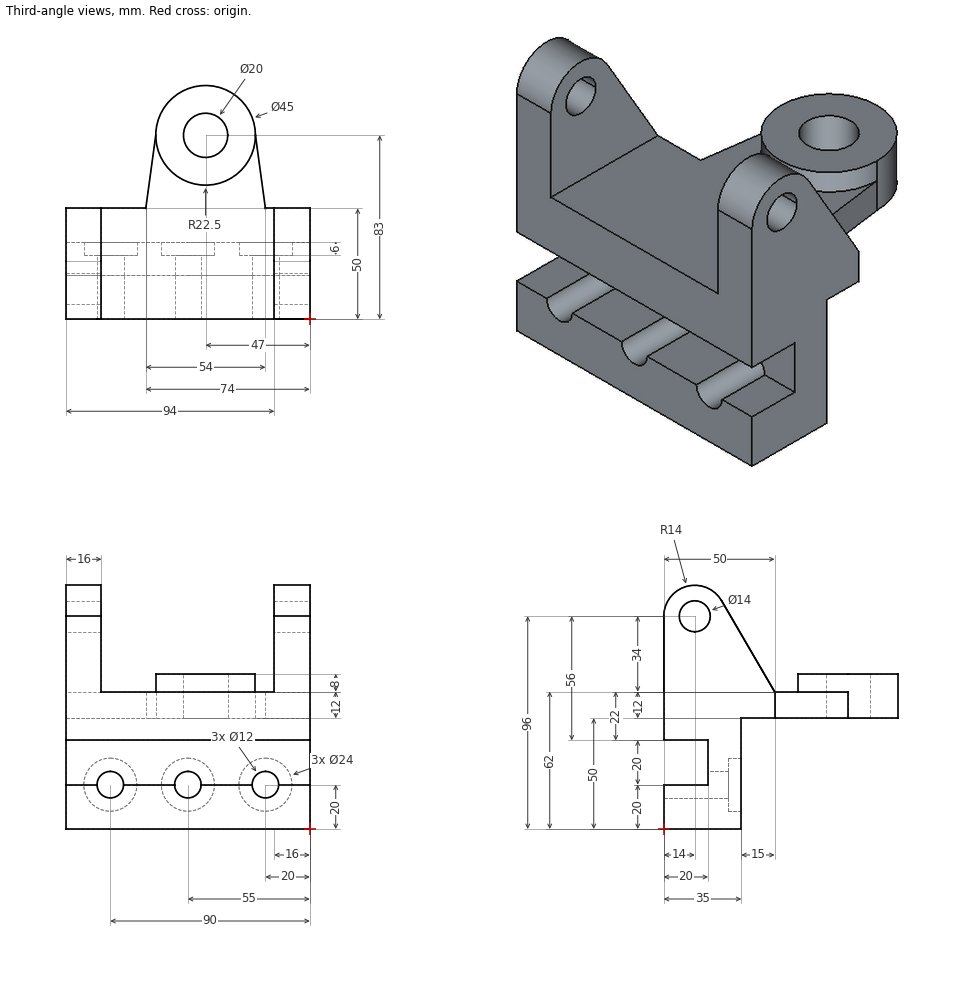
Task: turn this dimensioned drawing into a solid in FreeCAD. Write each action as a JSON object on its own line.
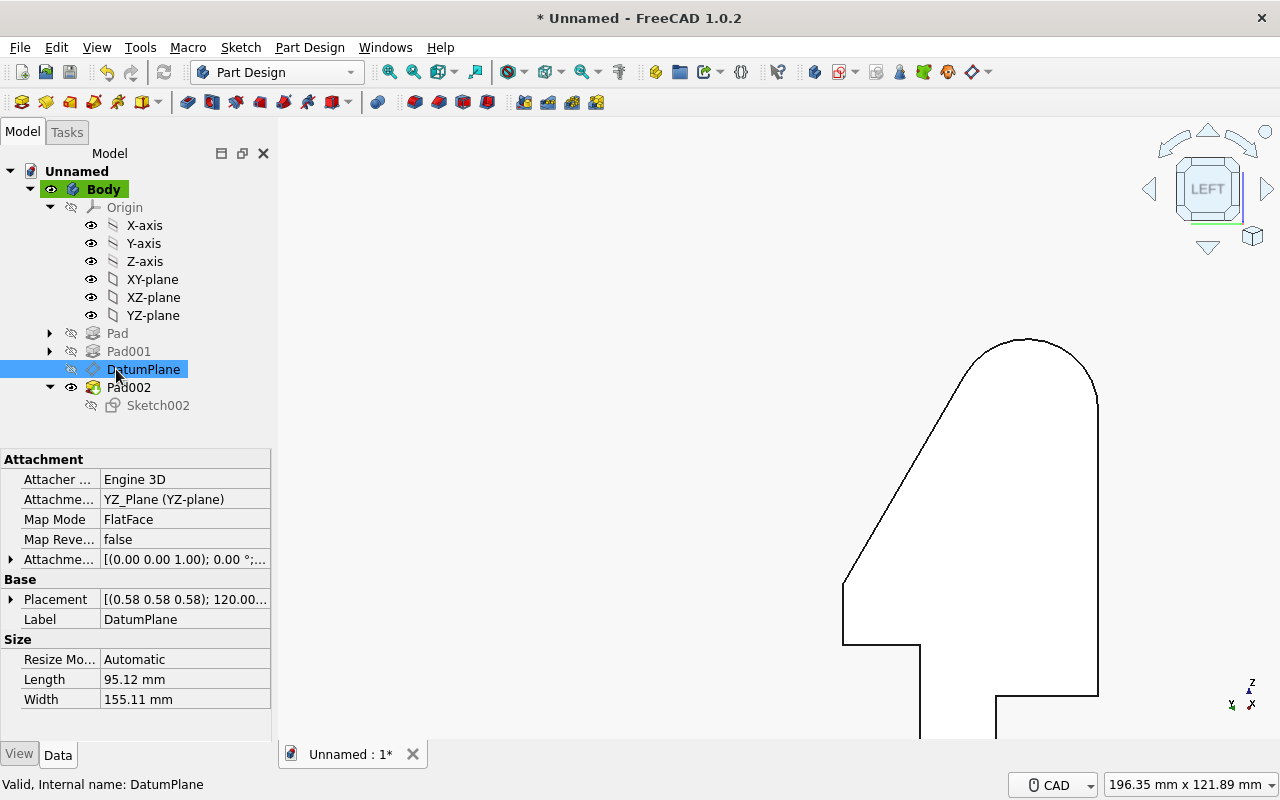
{"action": "left_click", "coordinate": [390, 72]}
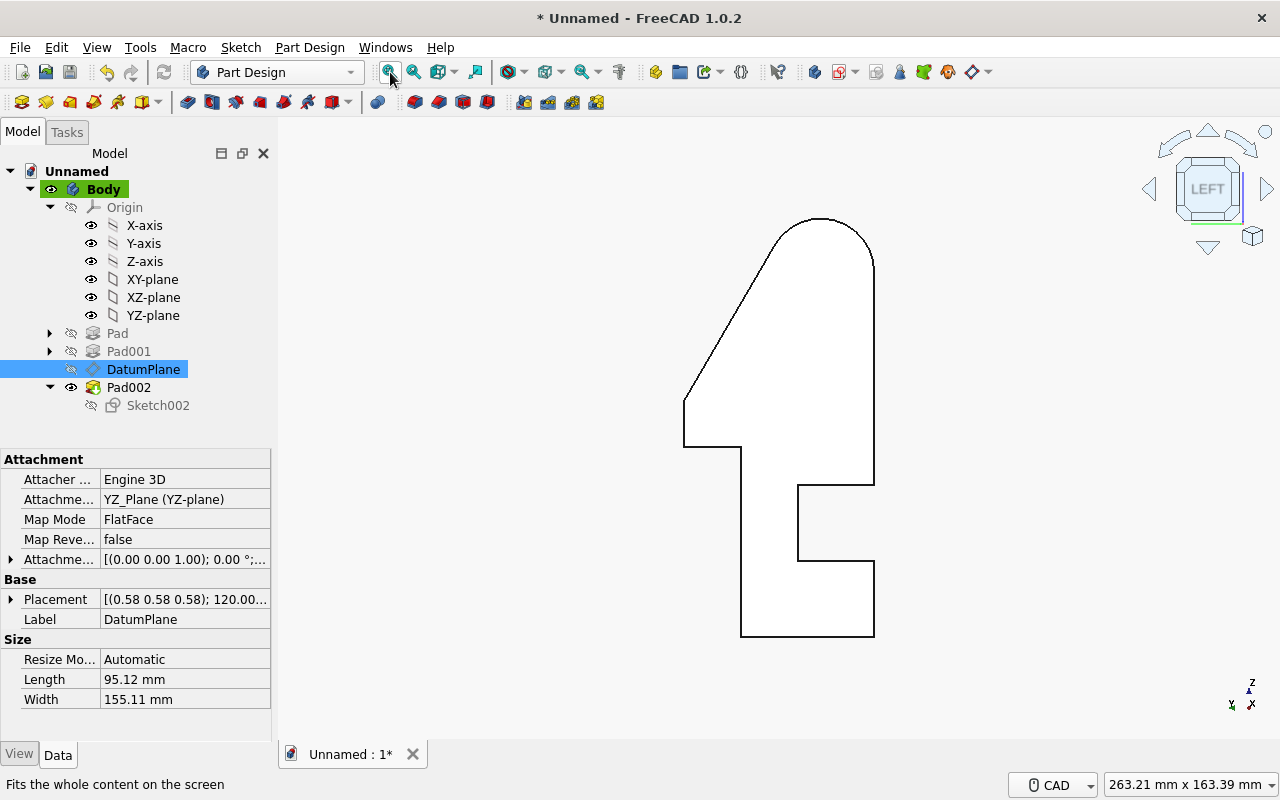
{"action": "key", "text": "0"}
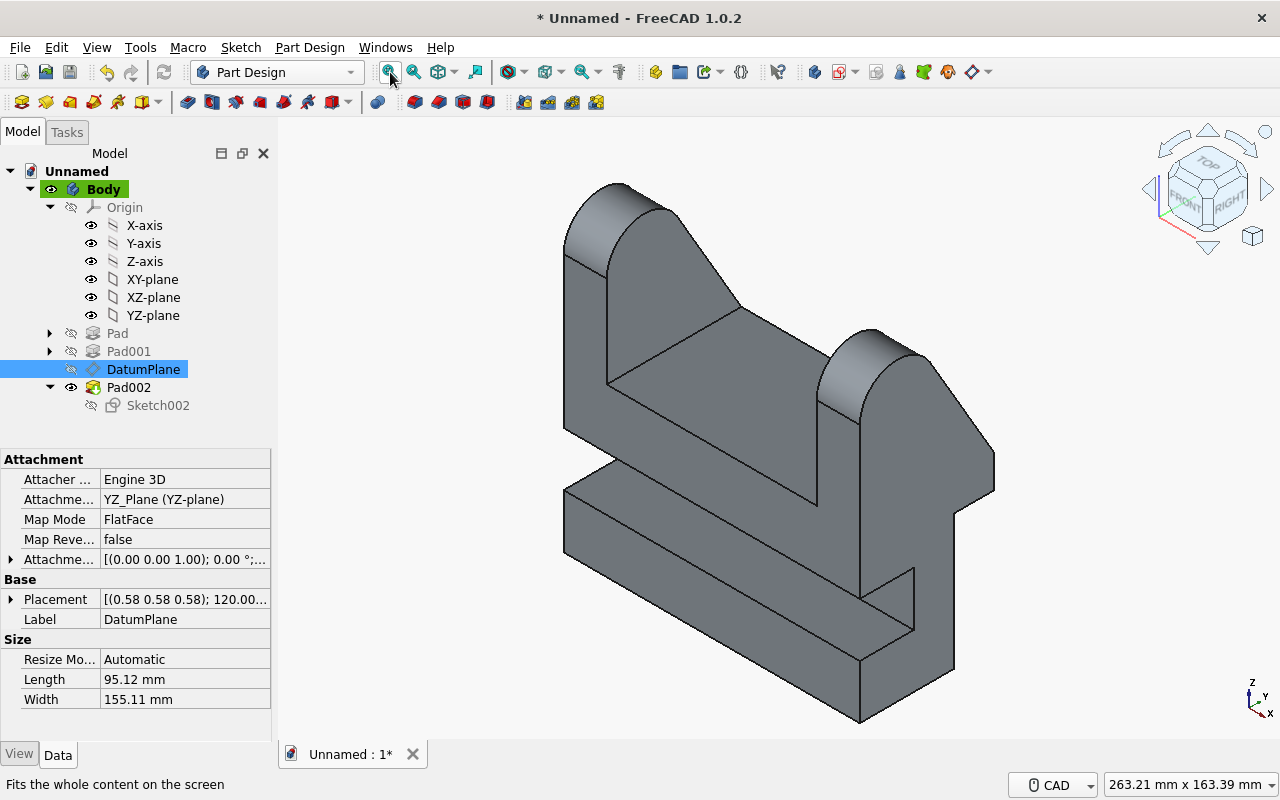
{"action": "left_click", "coordinate": [908, 475]}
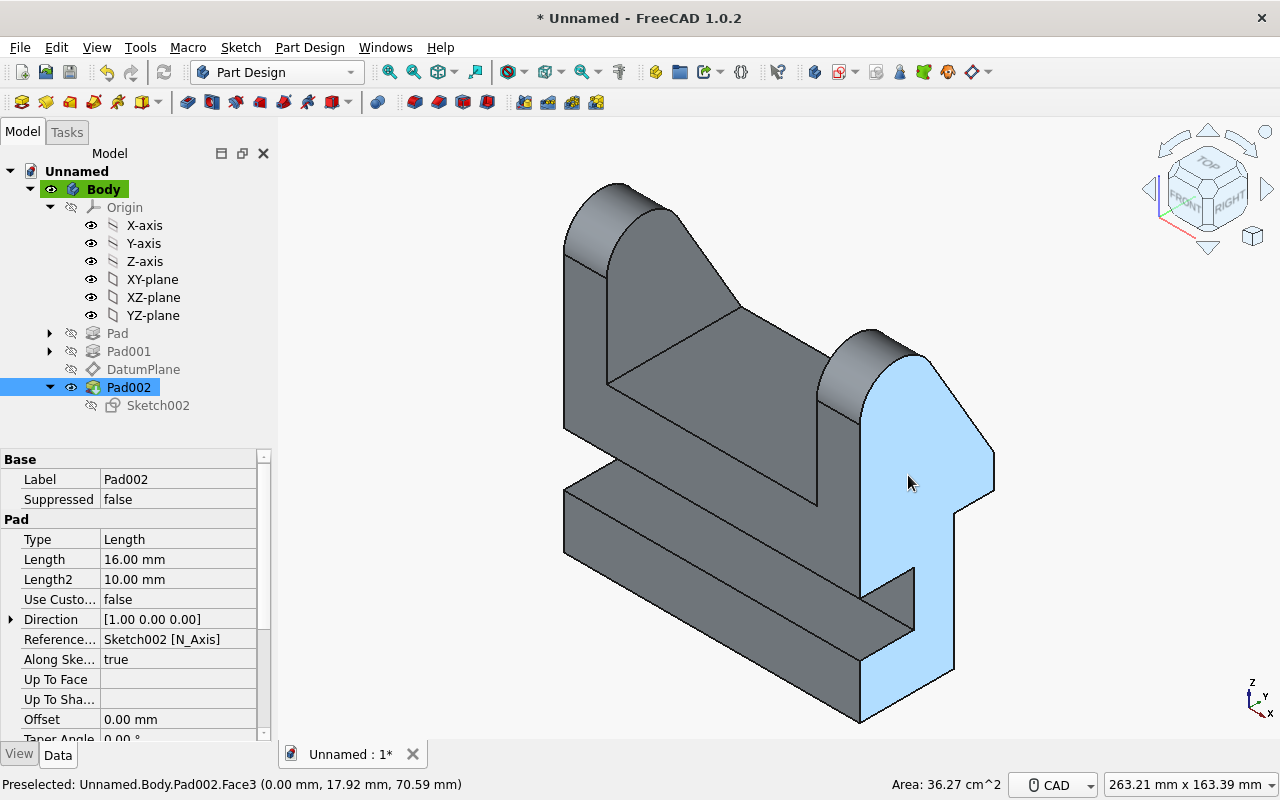
{"action": "left_click", "coordinate": [840, 72]}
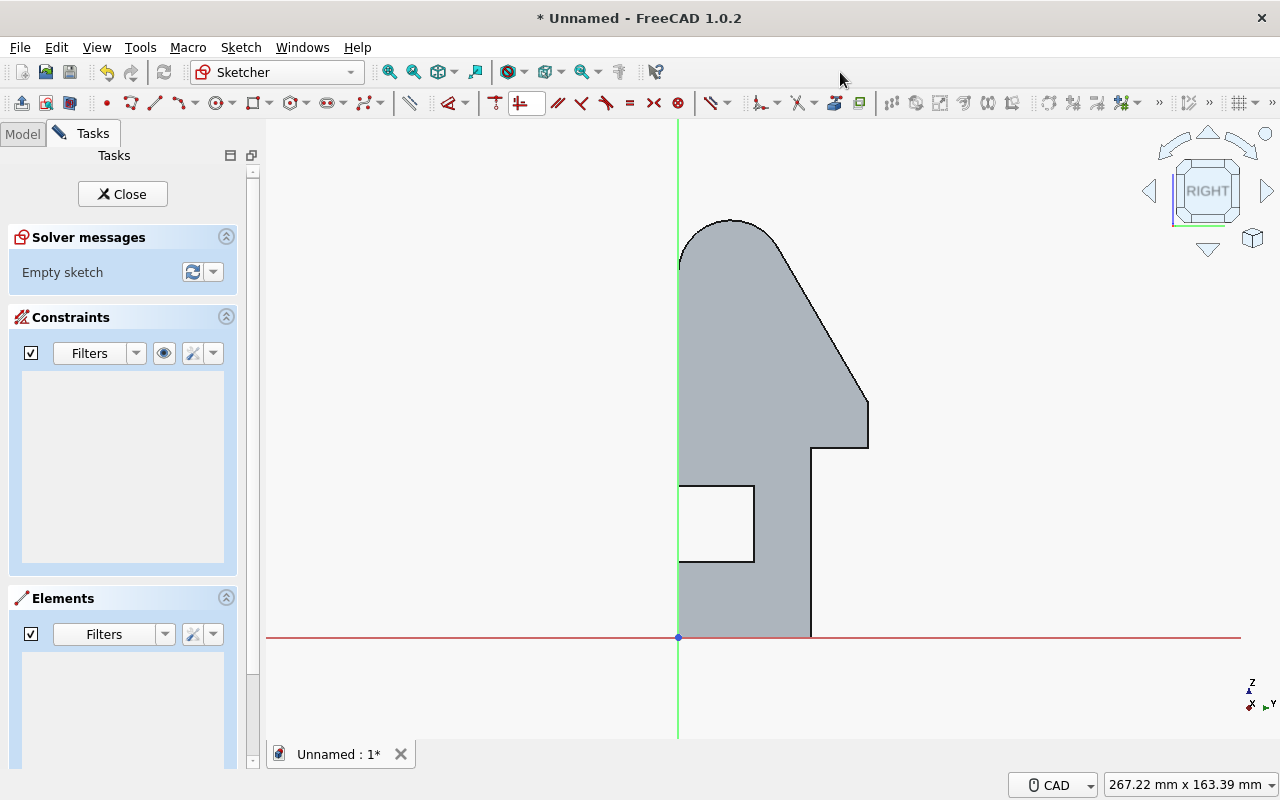
{"action": "scroll", "coordinate": [735, 249], "scroll_direction": "up", "scroll_amount": 10}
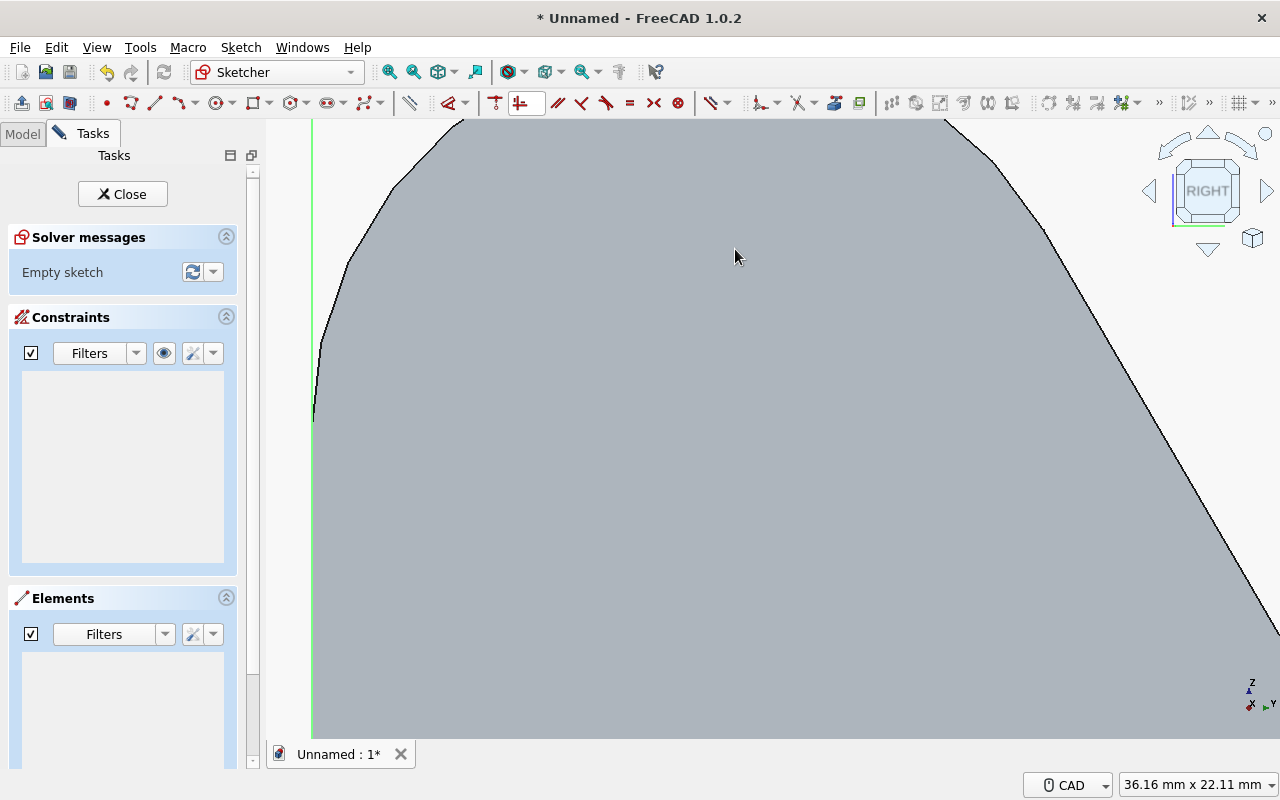
{"action": "key", "text": "g c"}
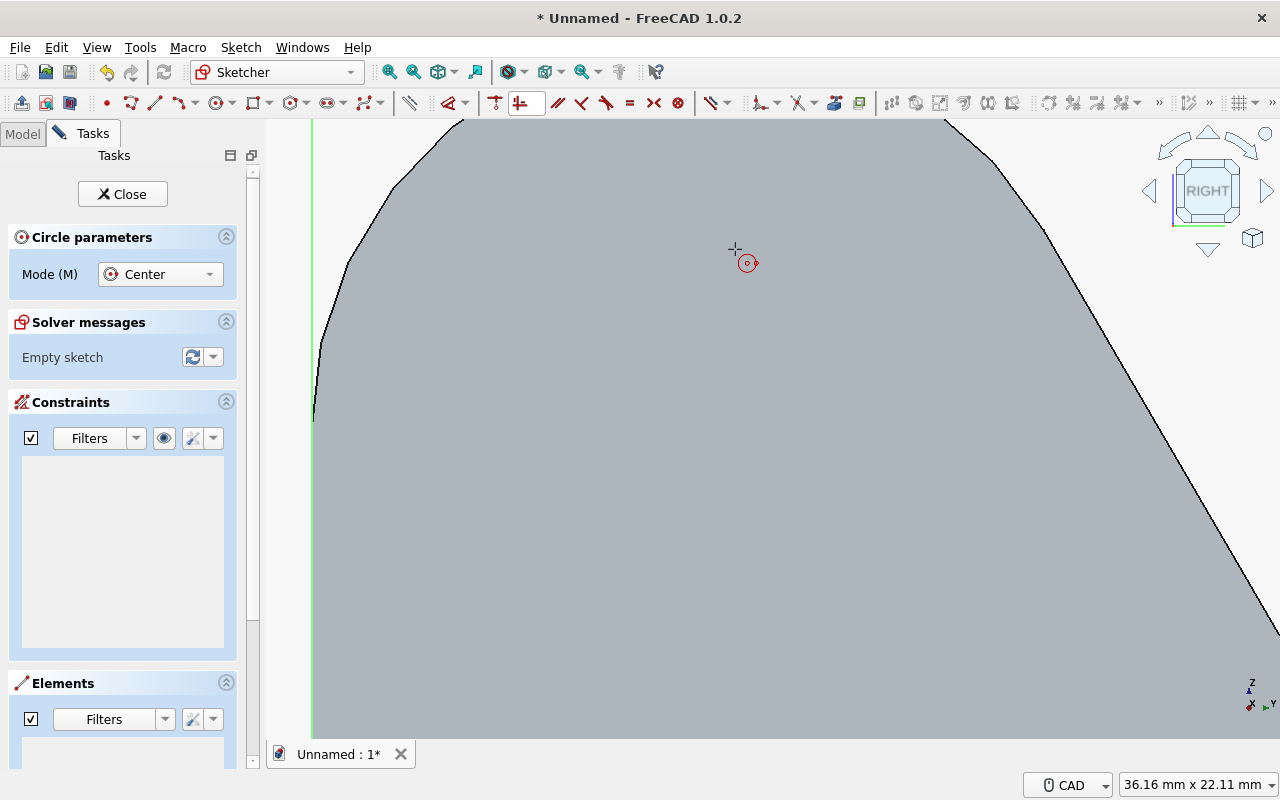
{"action": "left_click", "coordinate": [704, 428]}
{"action": "mouse_move", "coordinate": [843, 289]}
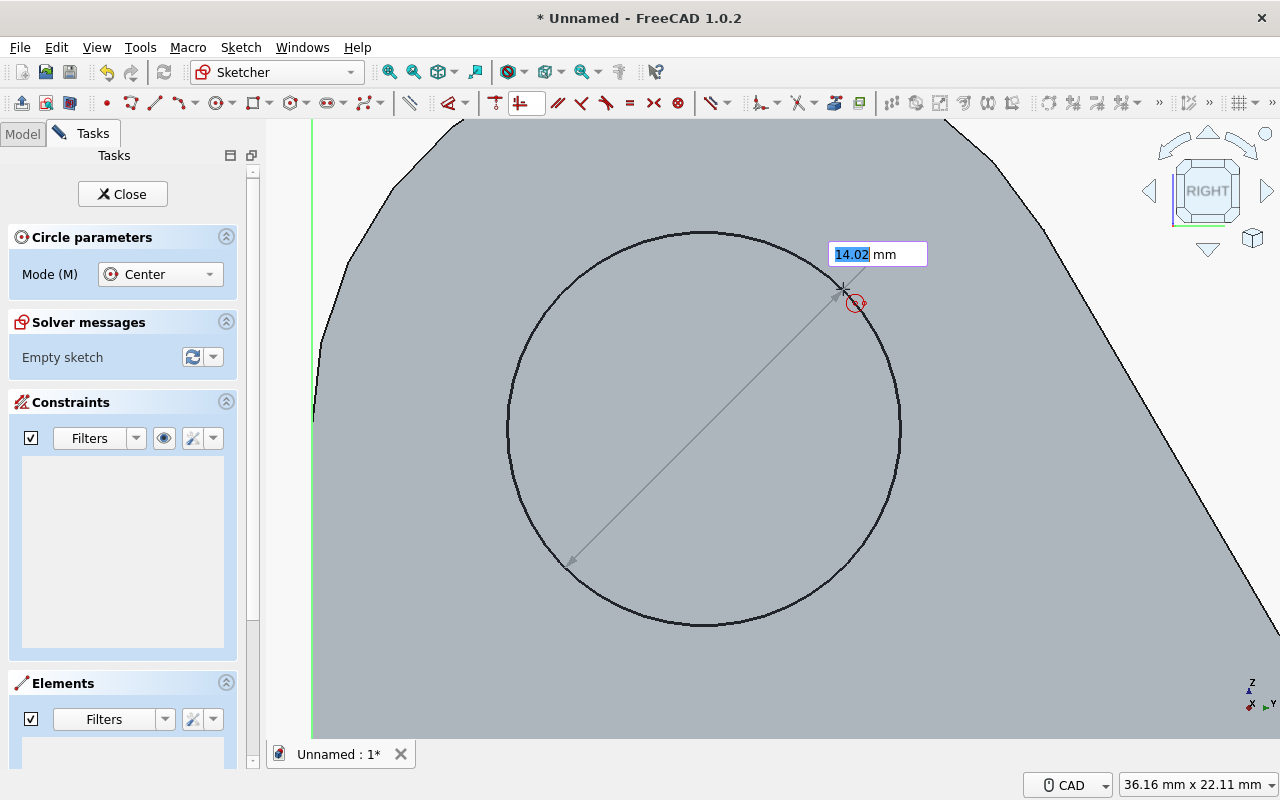
{"action": "type", "text": "14"}
{"action": "key", "text": "Return"}
{"action": "key", "text": "Escape"}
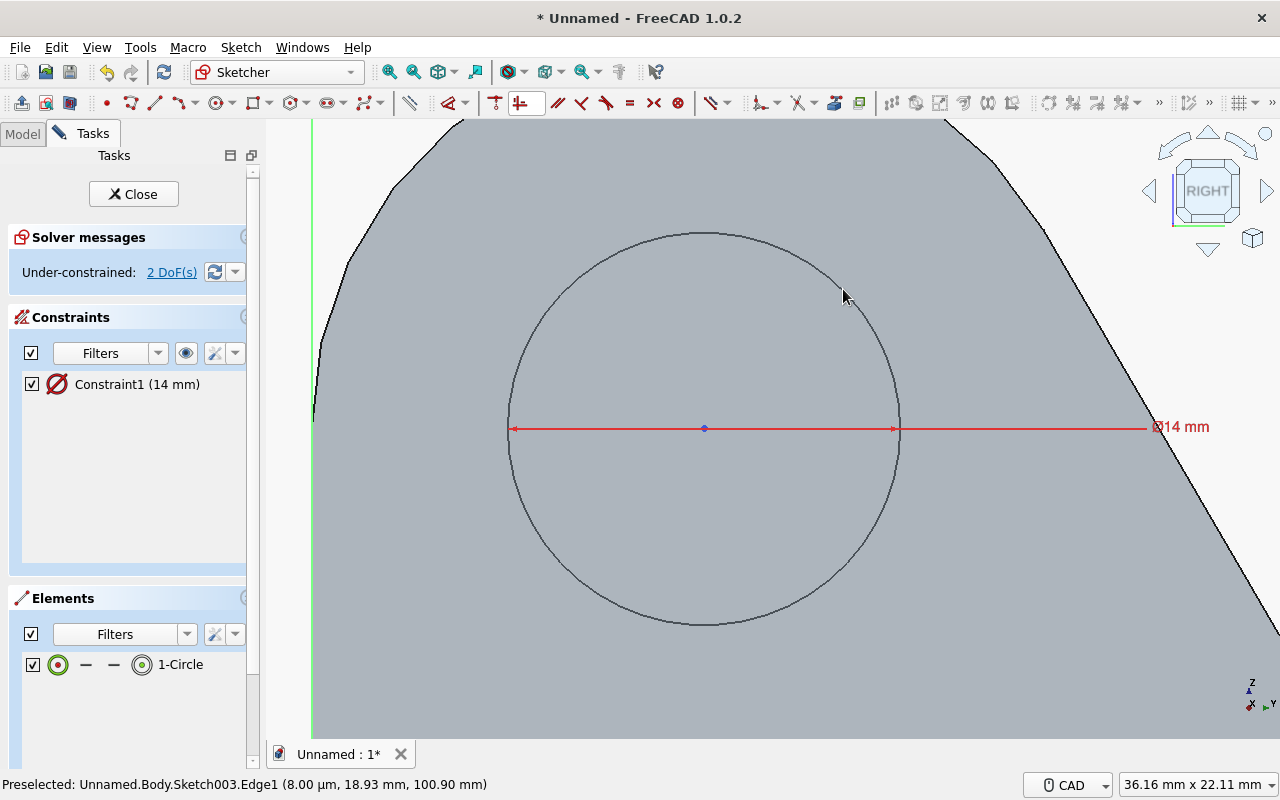
{"action": "left_click", "coordinate": [448, 104]}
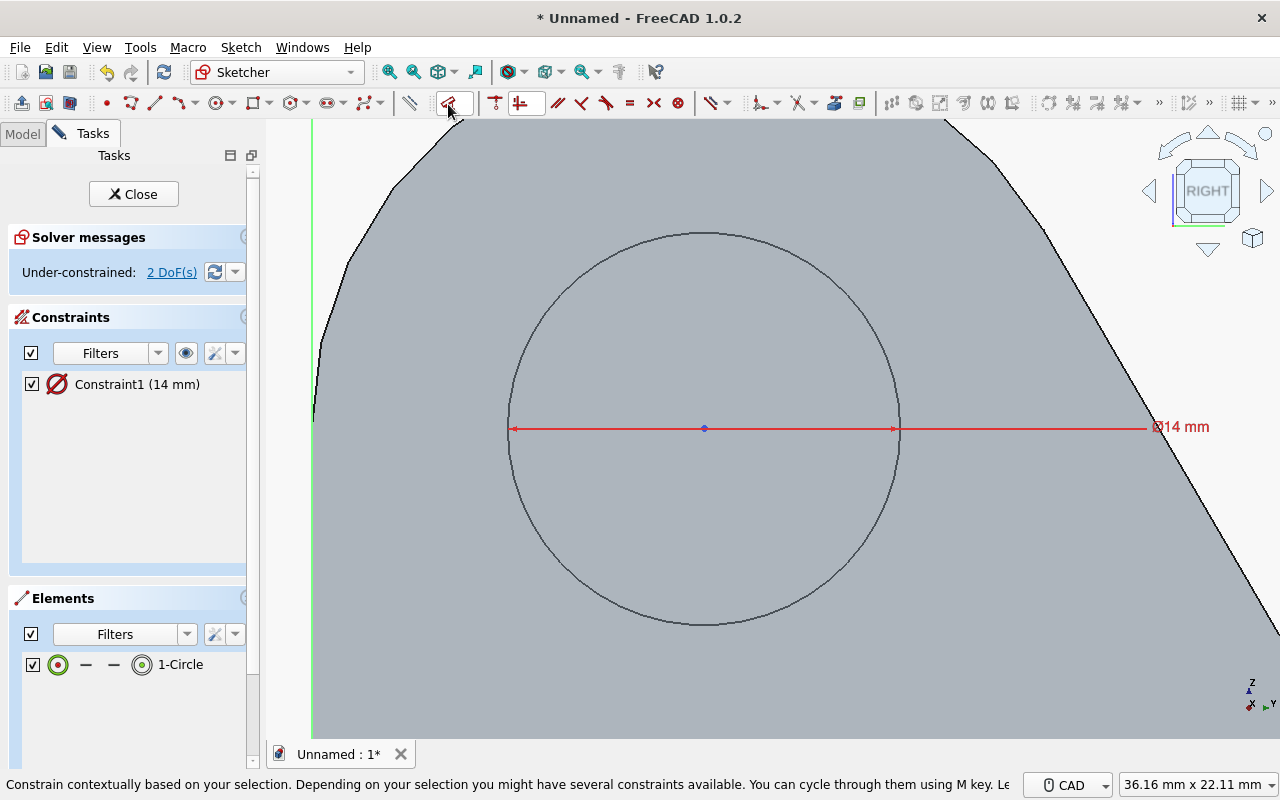
{"action": "left_click", "coordinate": [704, 429]}
{"action": "left_click", "coordinate": [418, 395]}